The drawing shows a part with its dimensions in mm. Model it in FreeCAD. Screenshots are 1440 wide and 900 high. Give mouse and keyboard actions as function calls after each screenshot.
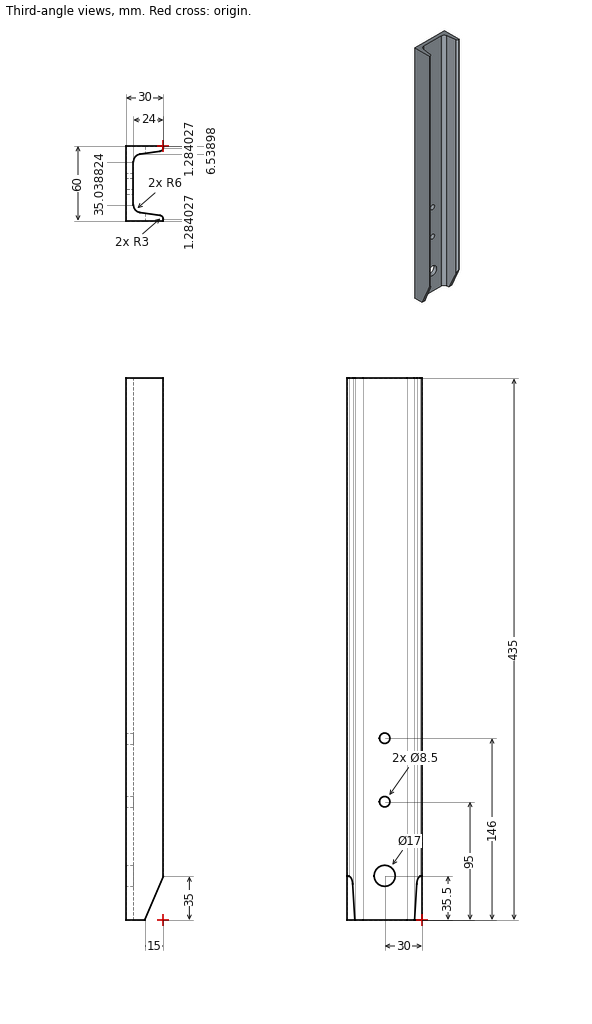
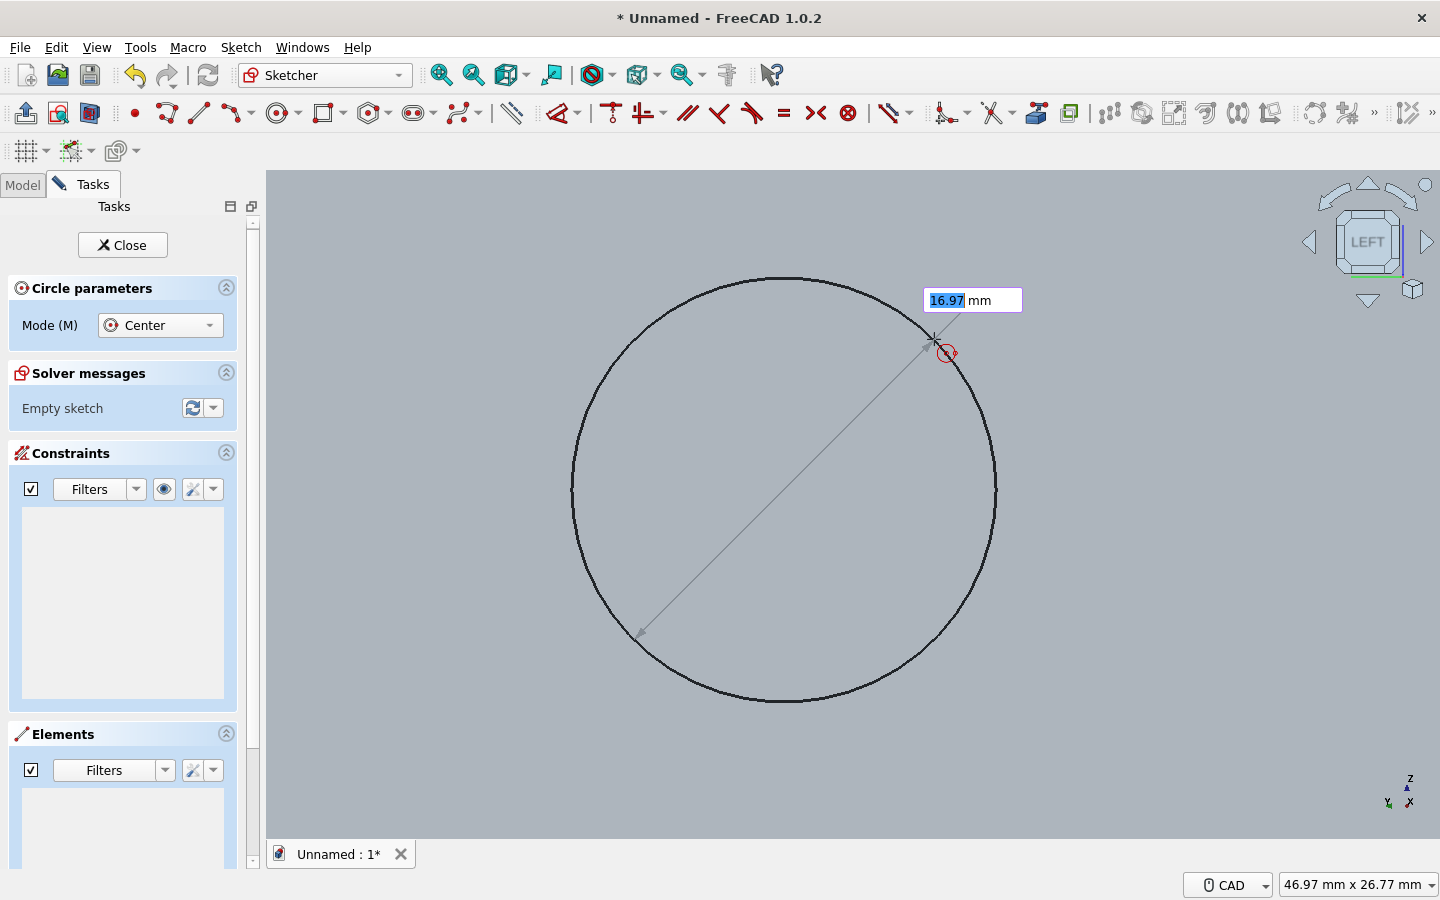
text(17)
key(Return)
key(Escape)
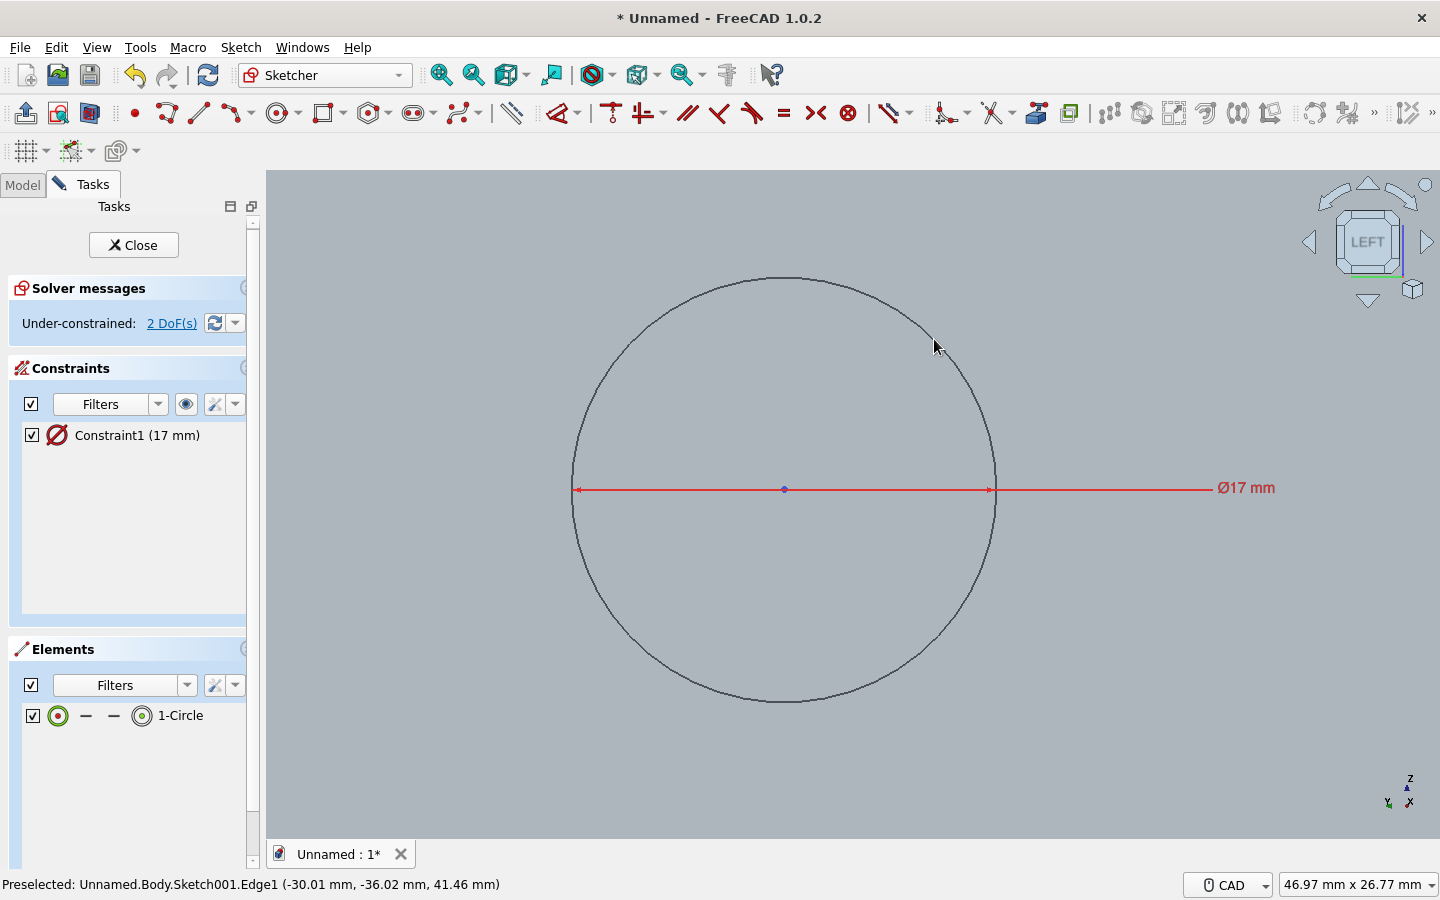
click(558, 114)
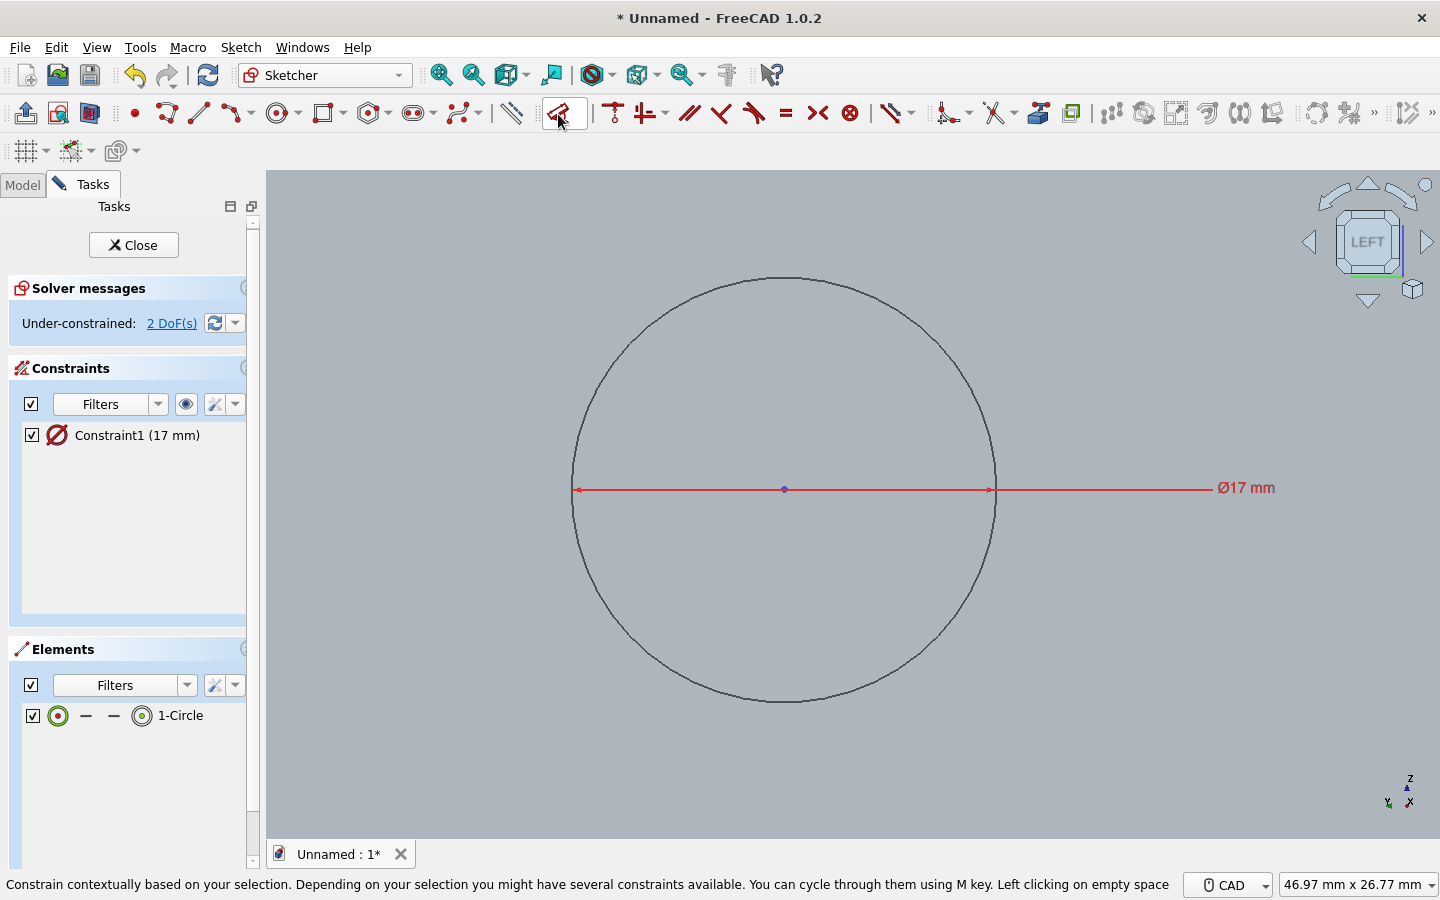
click(784, 490)
click(539, 456)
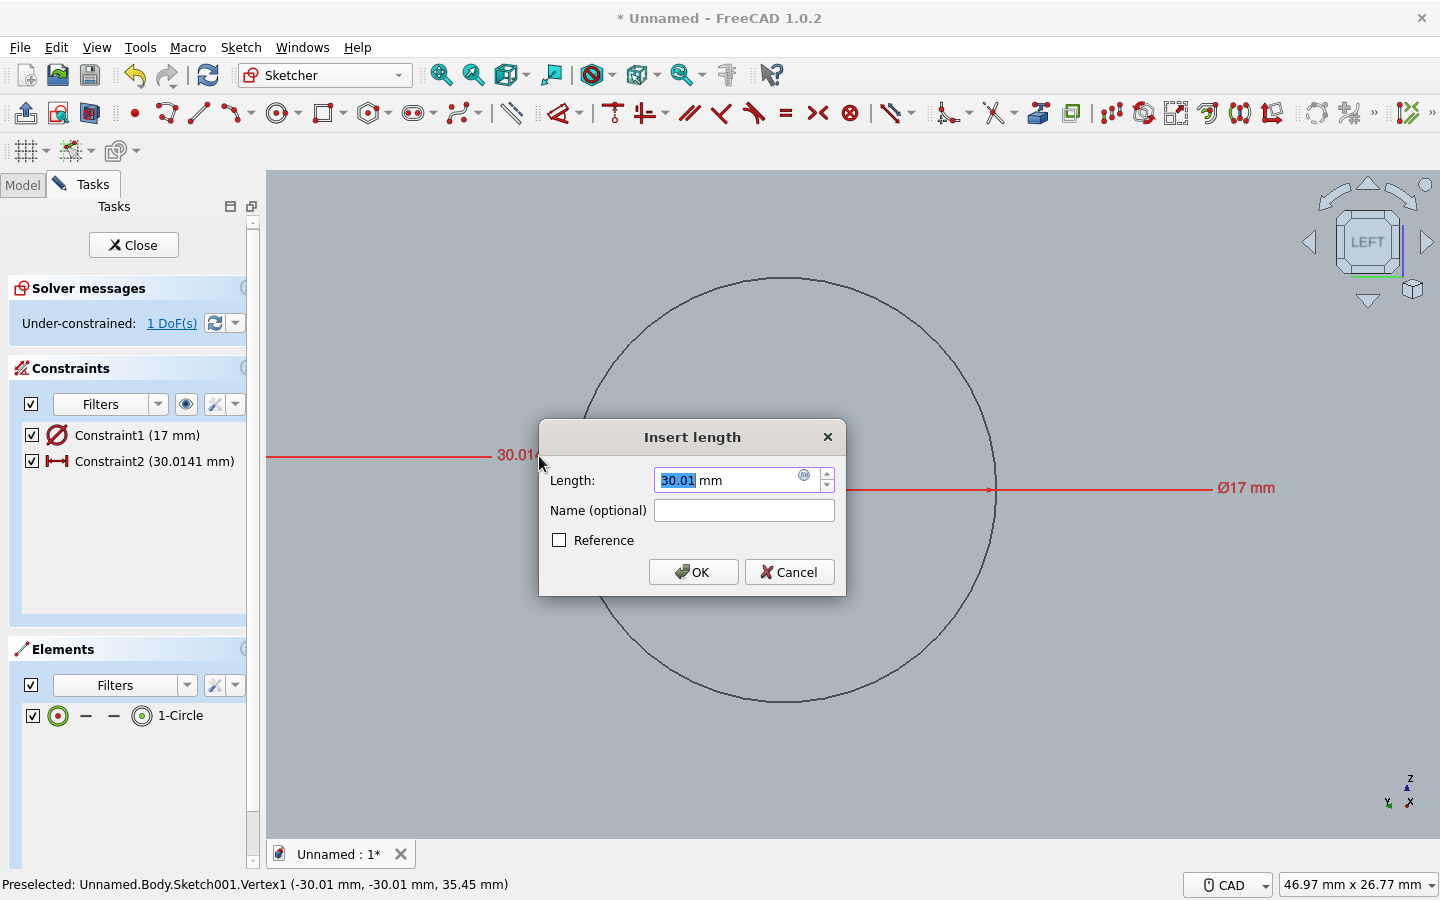
text(30)
key(Return)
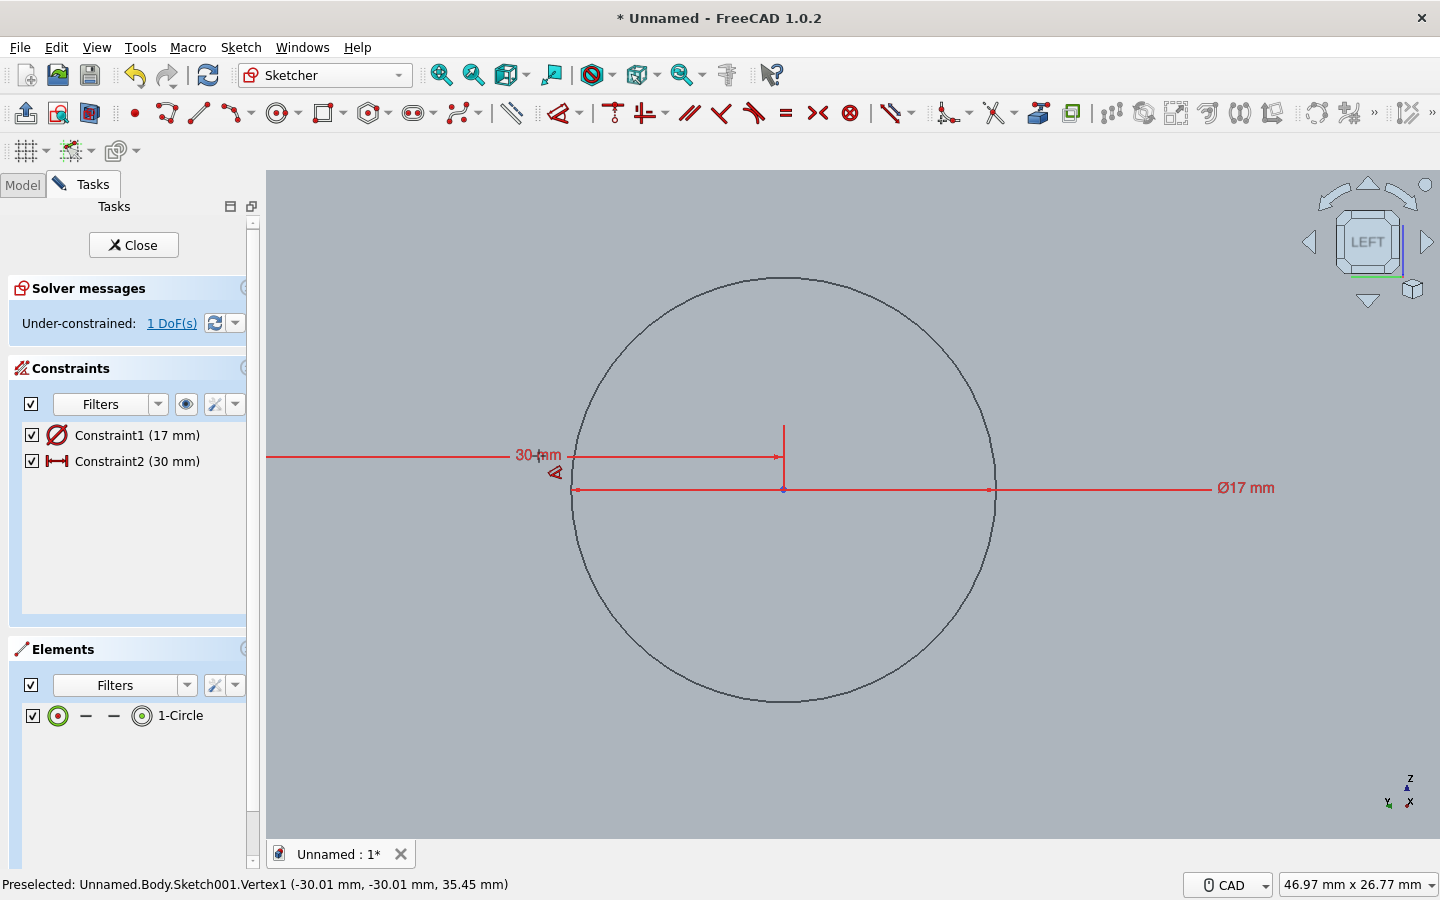
click(784, 490)
click(818, 651)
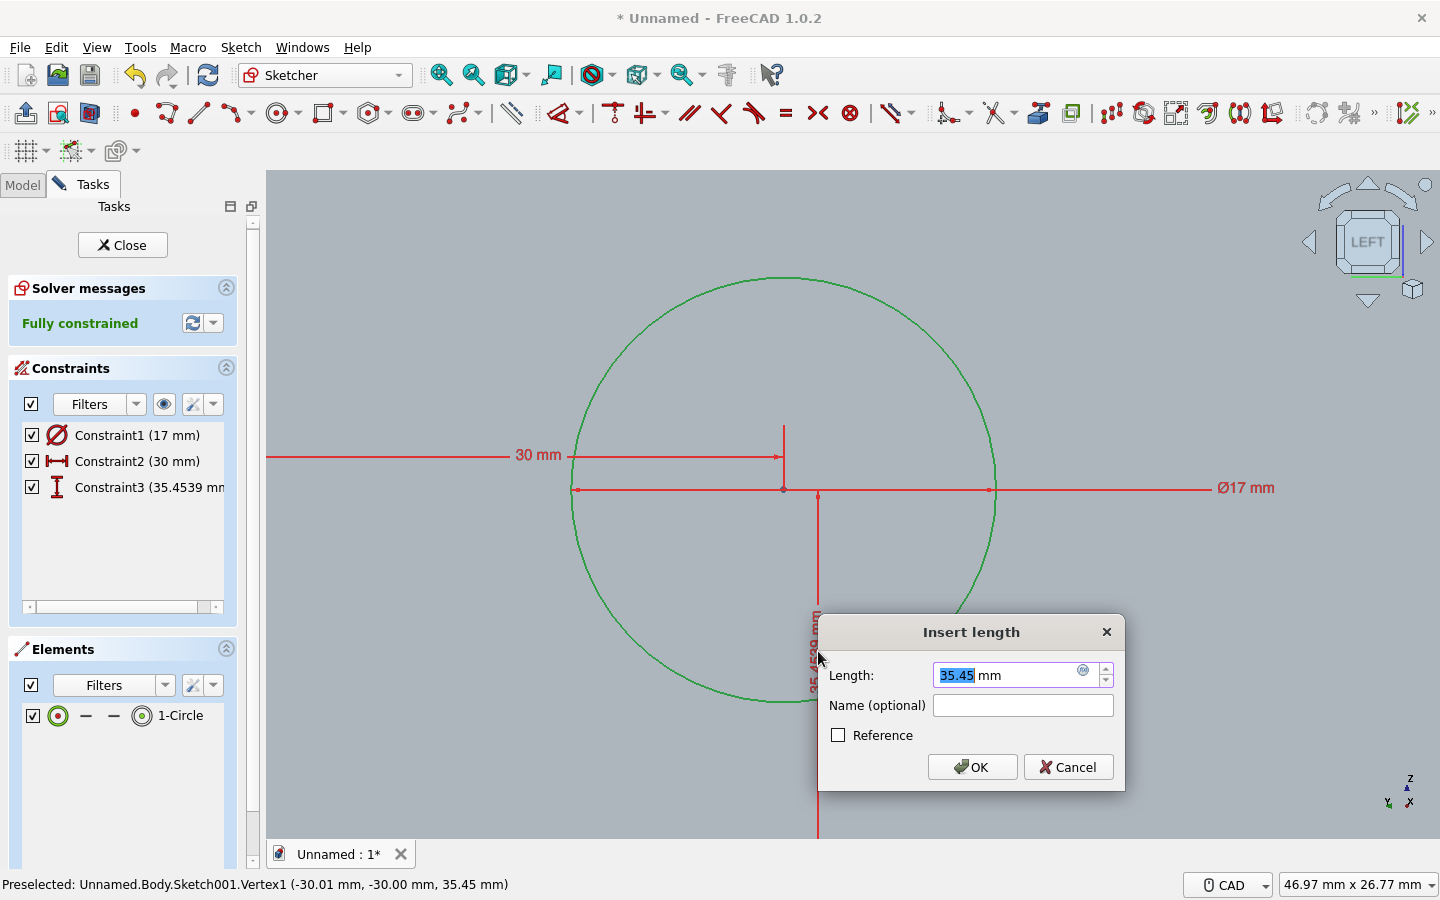
text(35.5)
key(Return)
key(Escape)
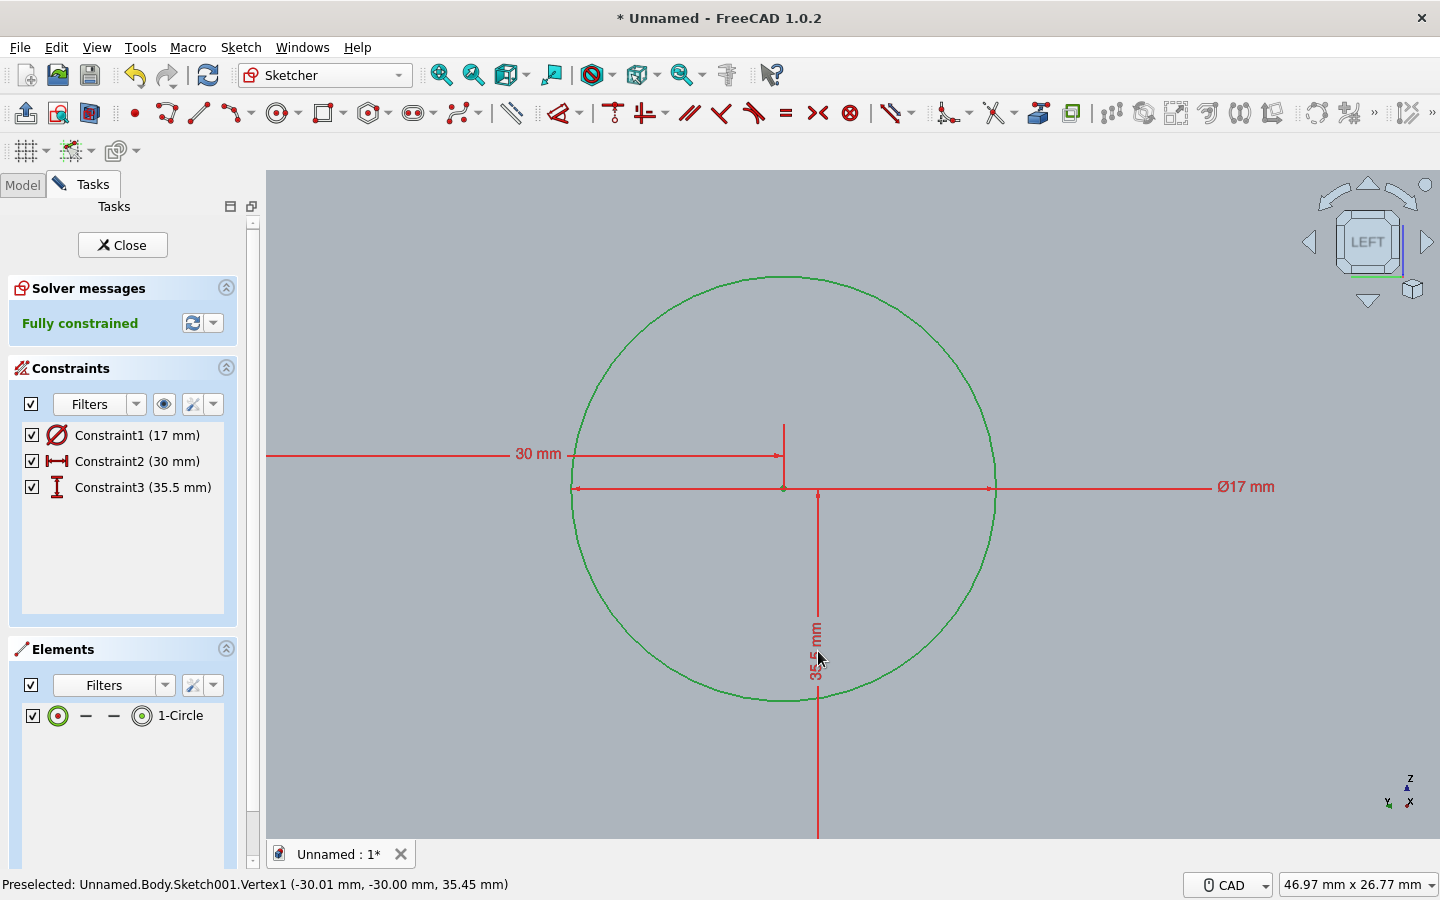
click(123, 245)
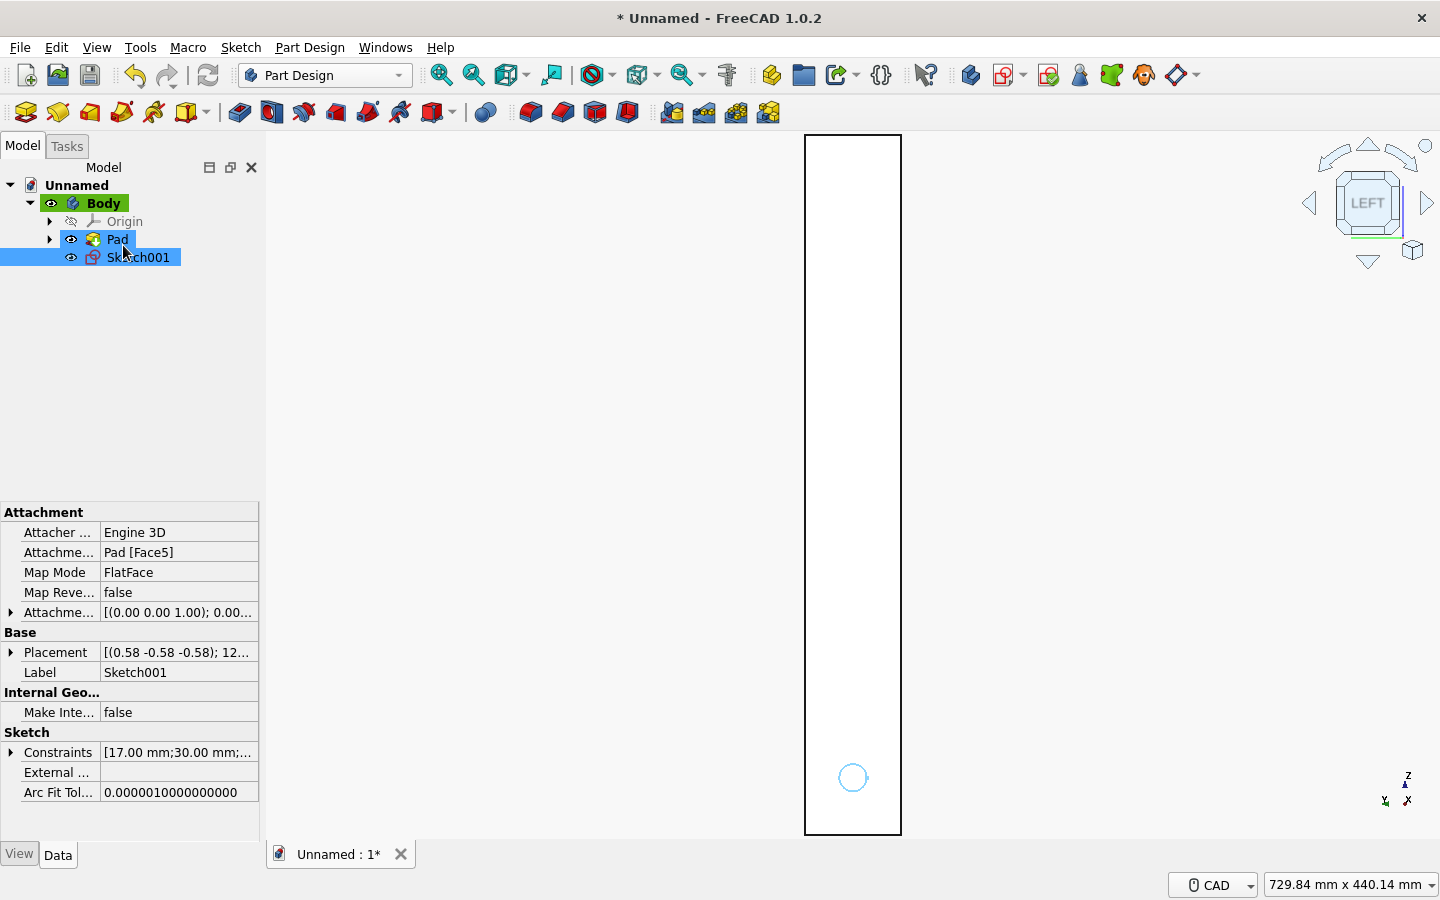
click(240, 112)